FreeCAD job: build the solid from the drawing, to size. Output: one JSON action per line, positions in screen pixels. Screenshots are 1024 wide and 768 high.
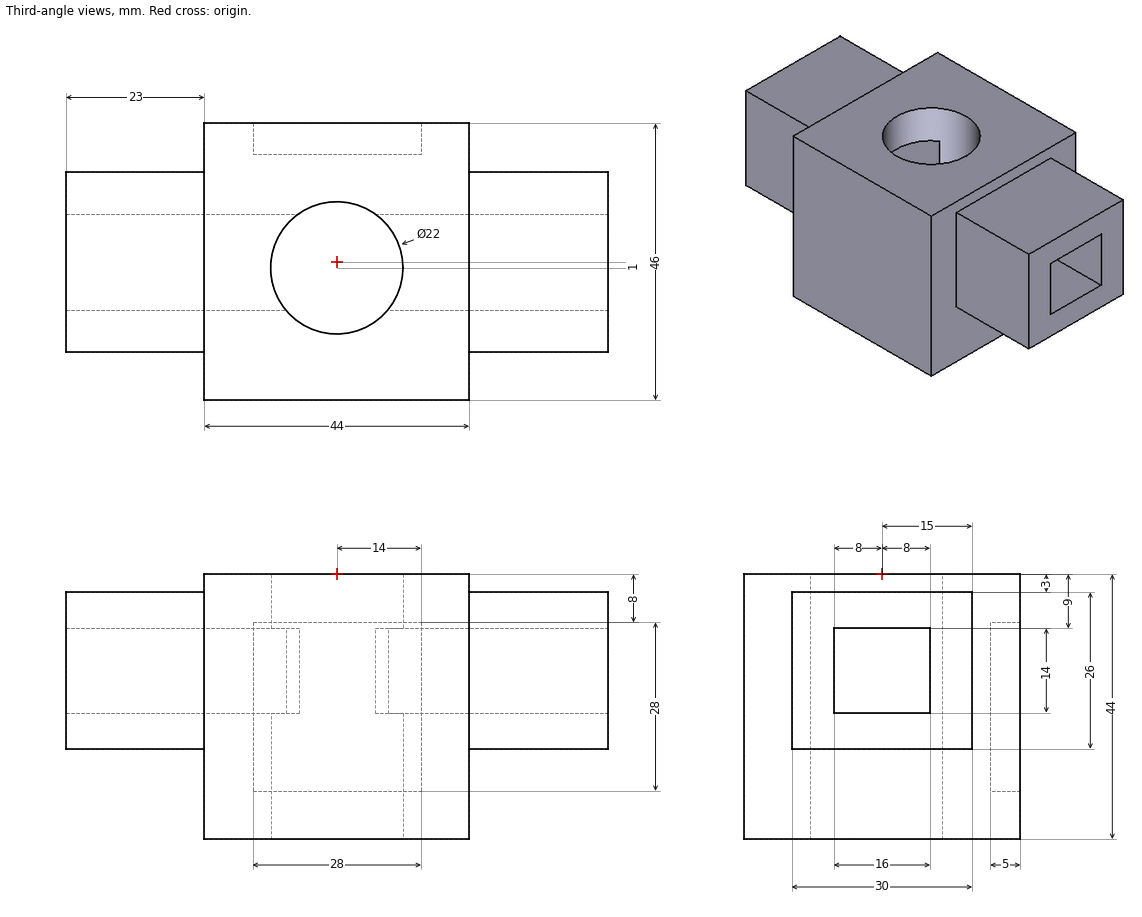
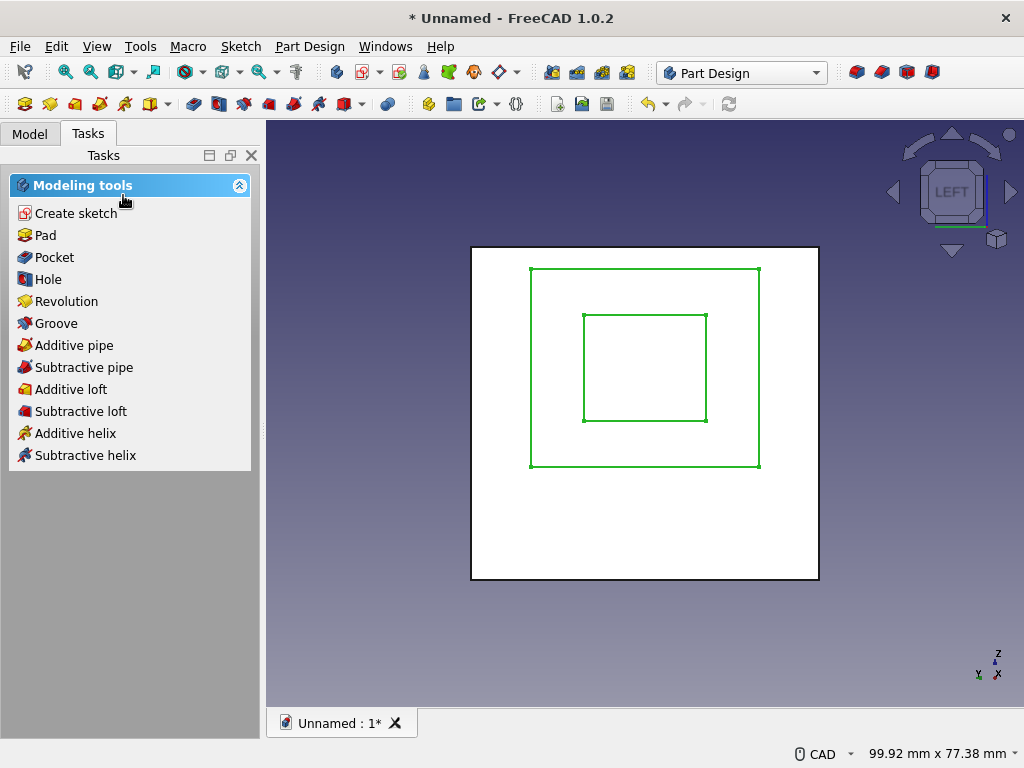
{"action": "left_click", "coordinate": [25, 104]}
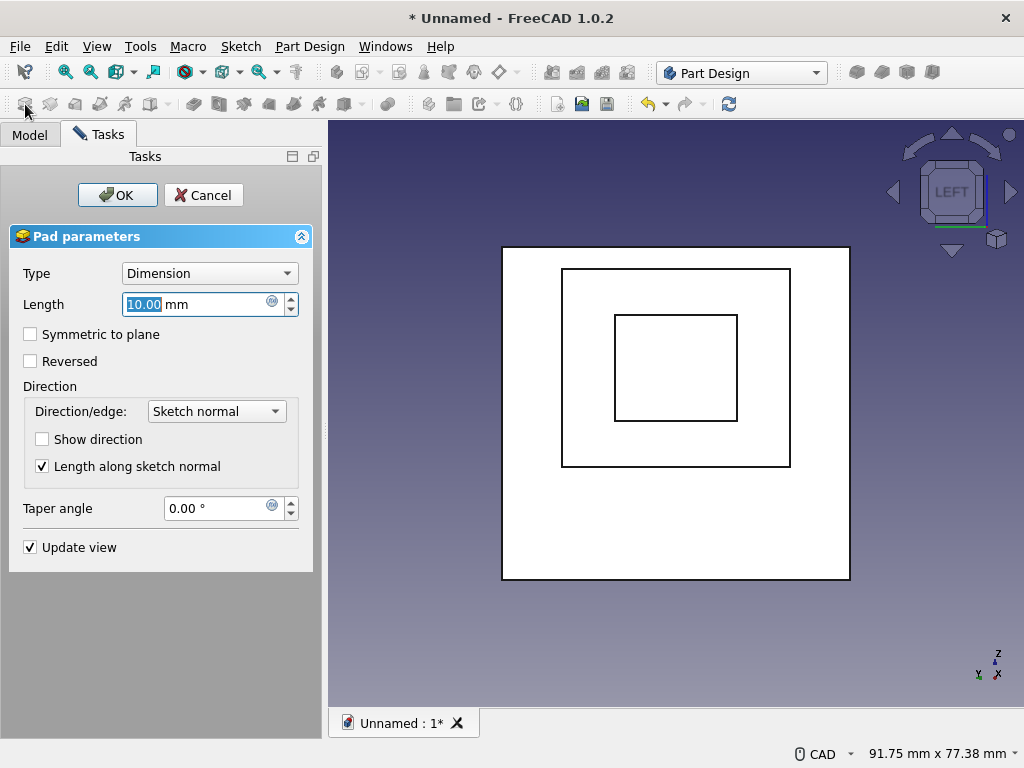
{"action": "type", "text": "23"}
{"action": "key", "text": "Tab"}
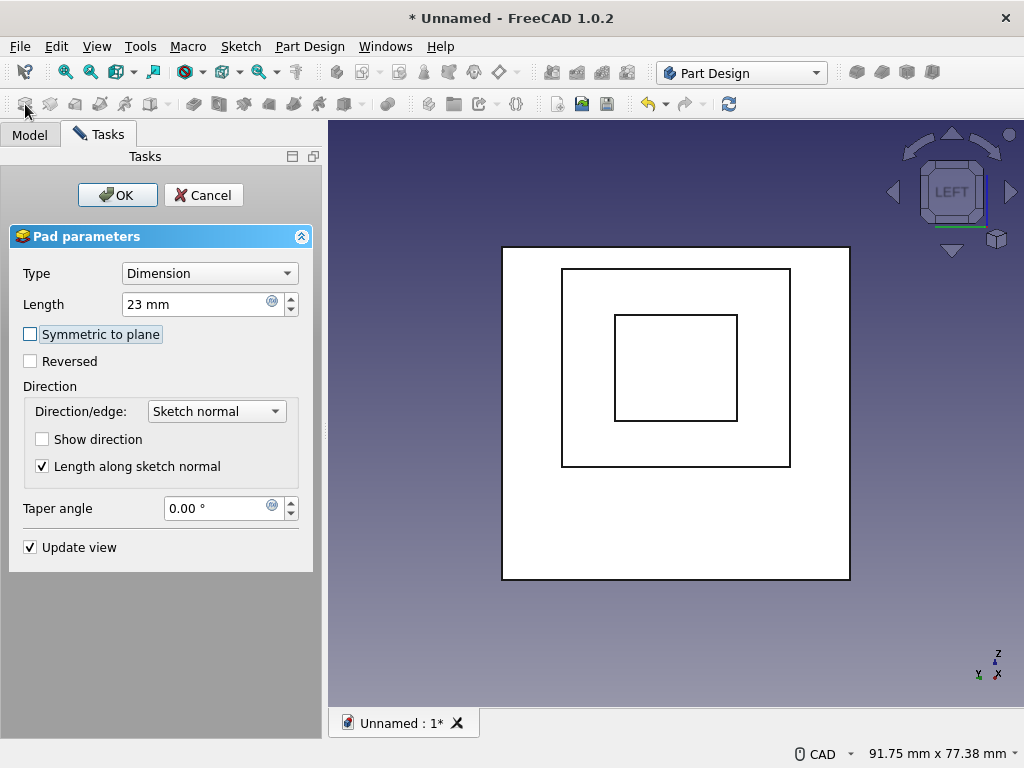
{"action": "left_click", "coordinate": [118, 195]}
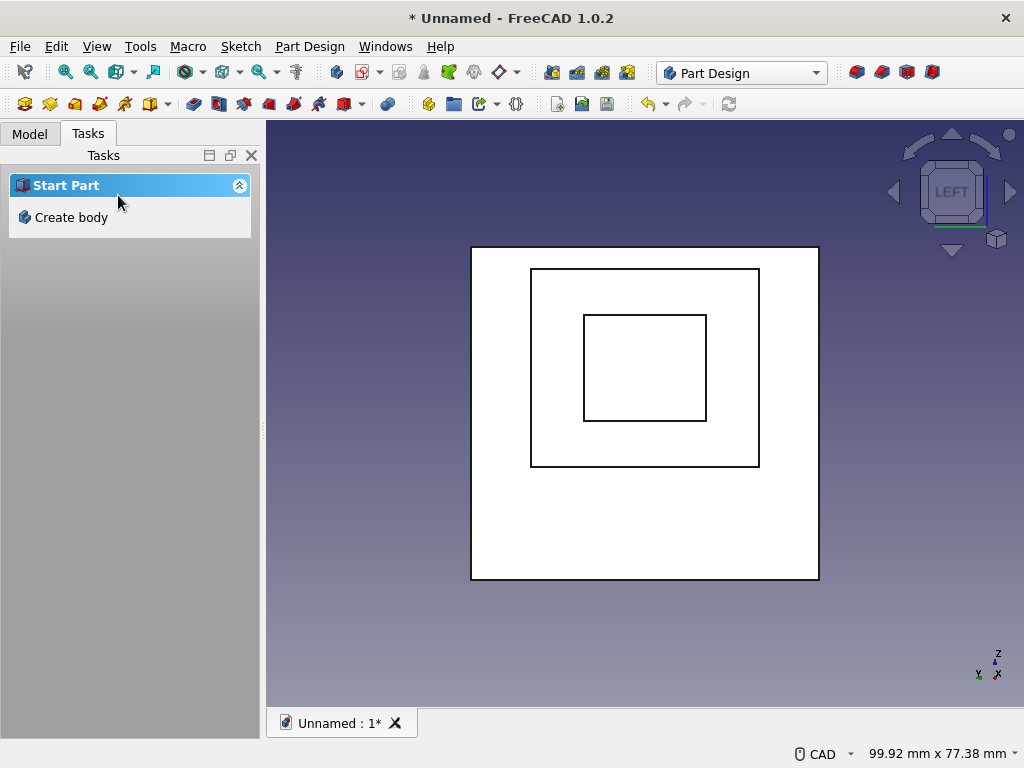
{"action": "left_click", "coordinate": [30, 134]}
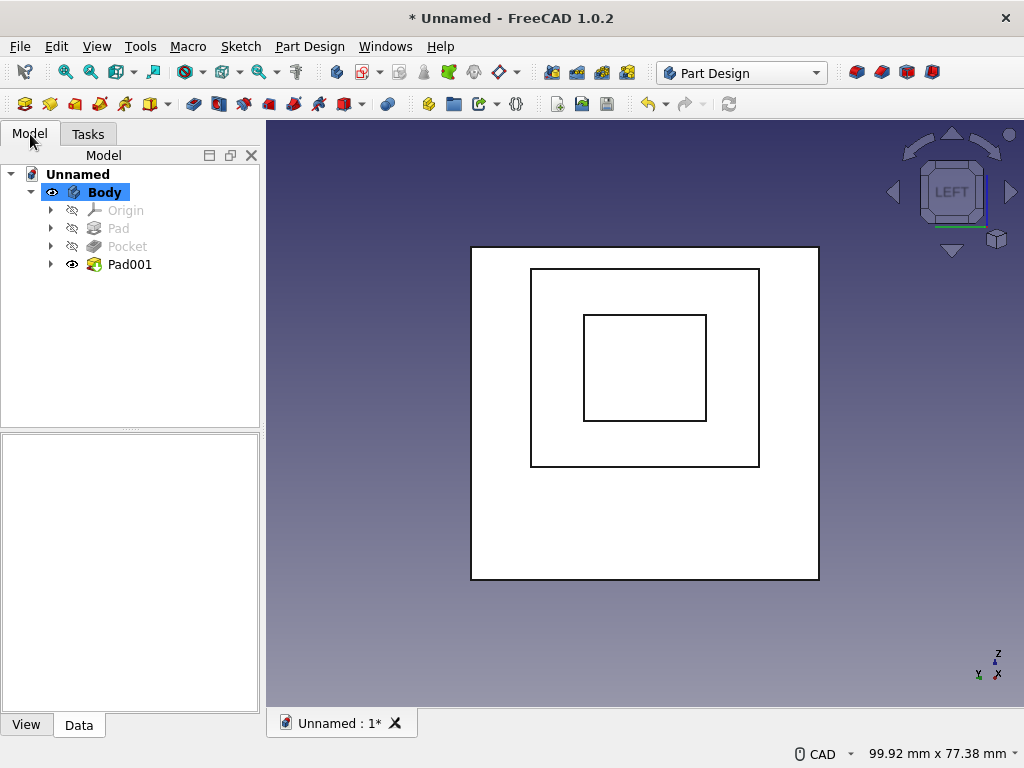
{"action": "left_click", "coordinate": [117, 264]}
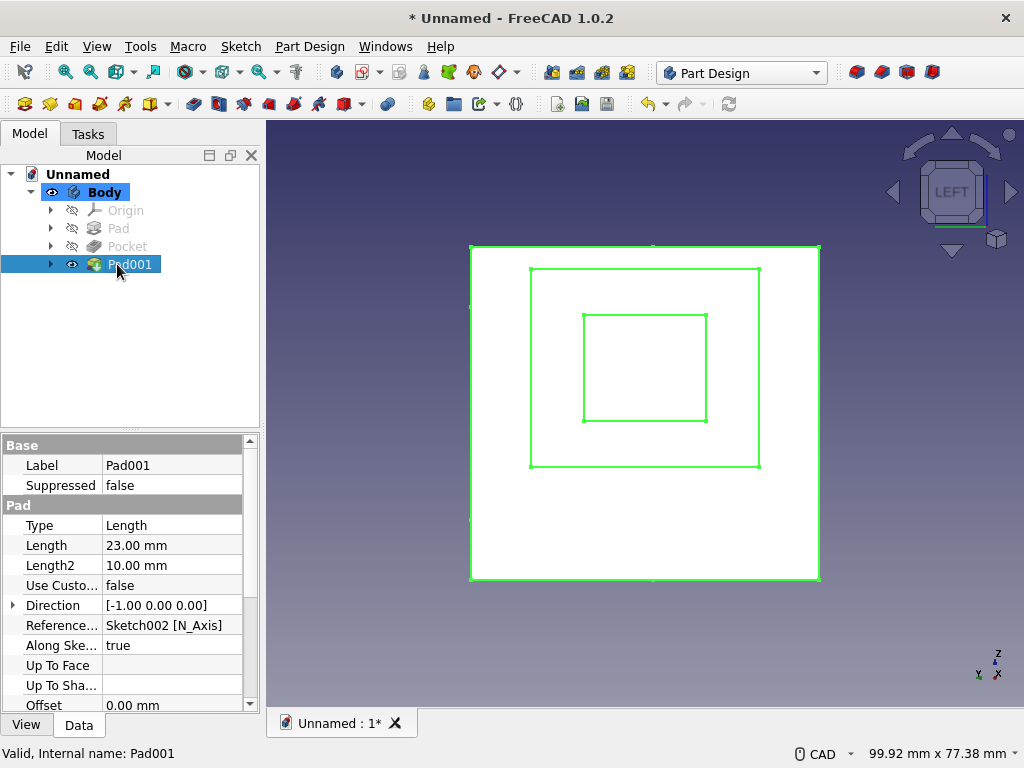
{"action": "left_click", "coordinate": [552, 72]}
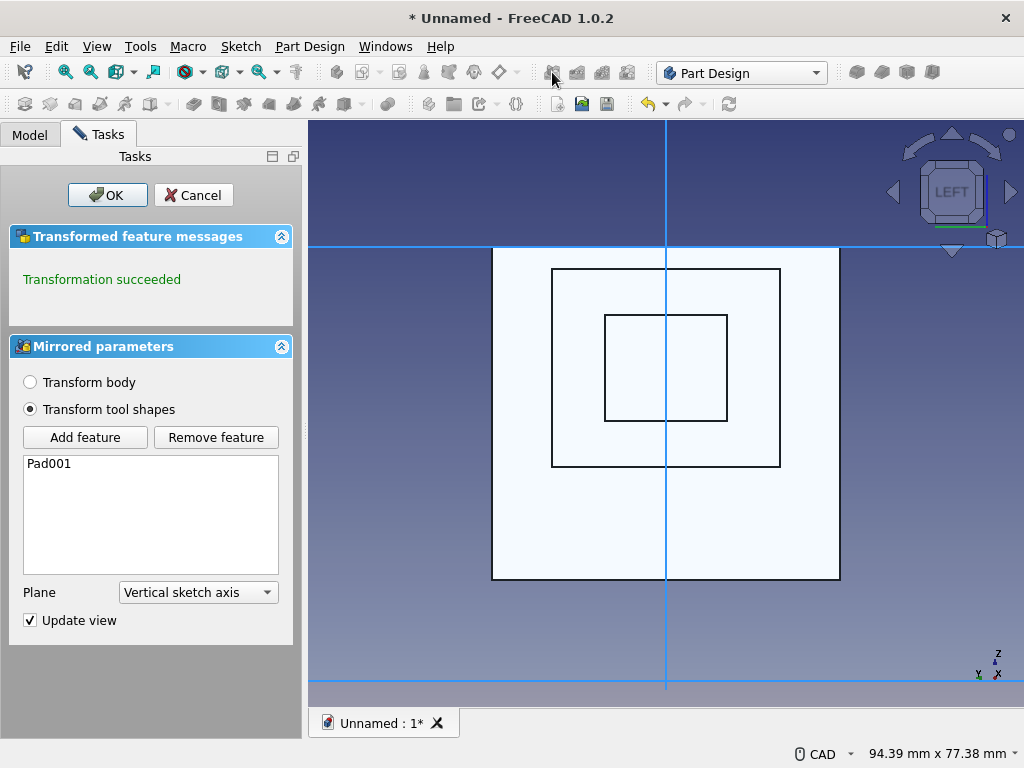
{"action": "left_click", "coordinate": [199, 592]}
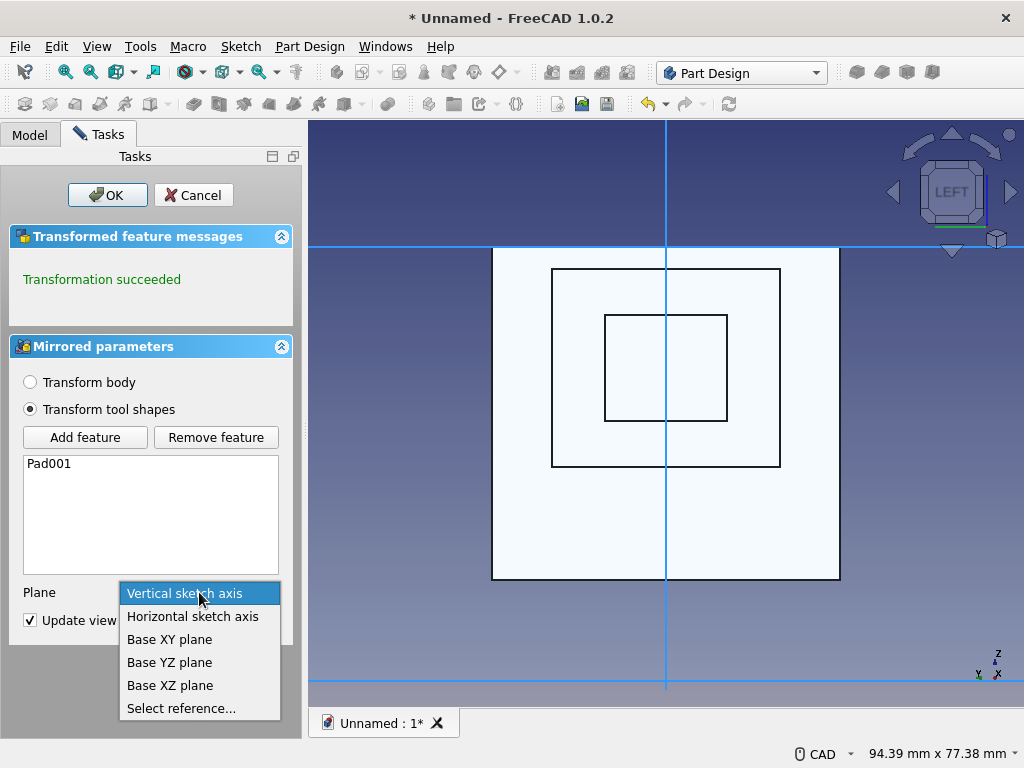
{"action": "left_click", "coordinate": [198, 662]}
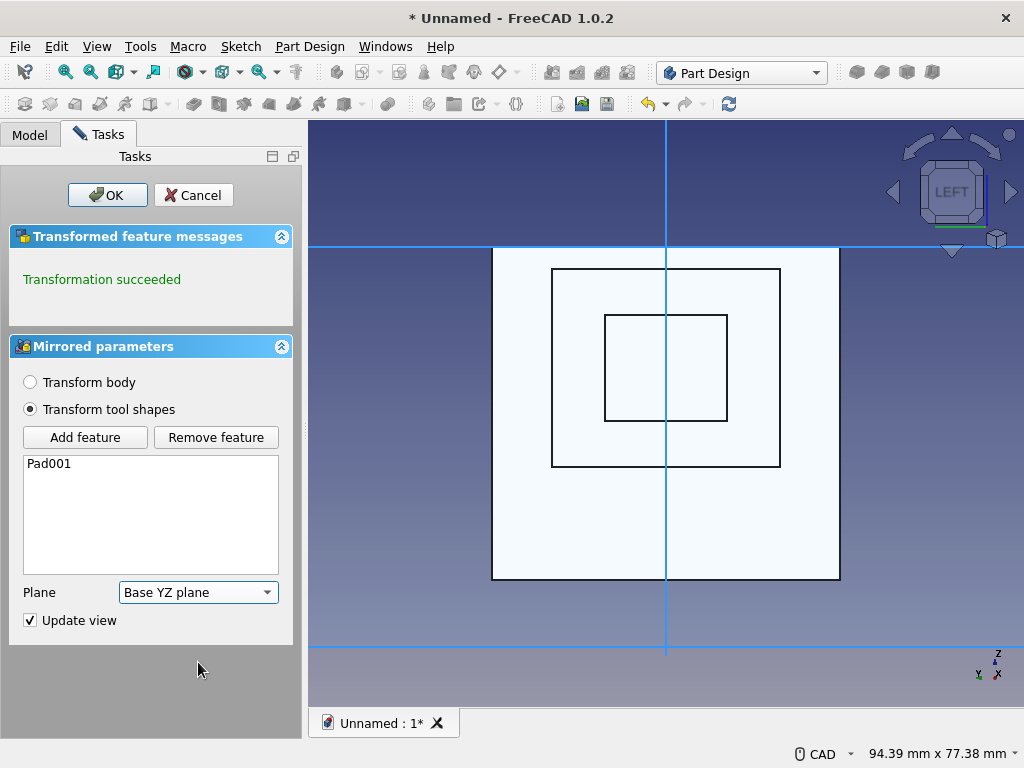
{"action": "left_click", "coordinate": [108, 195]}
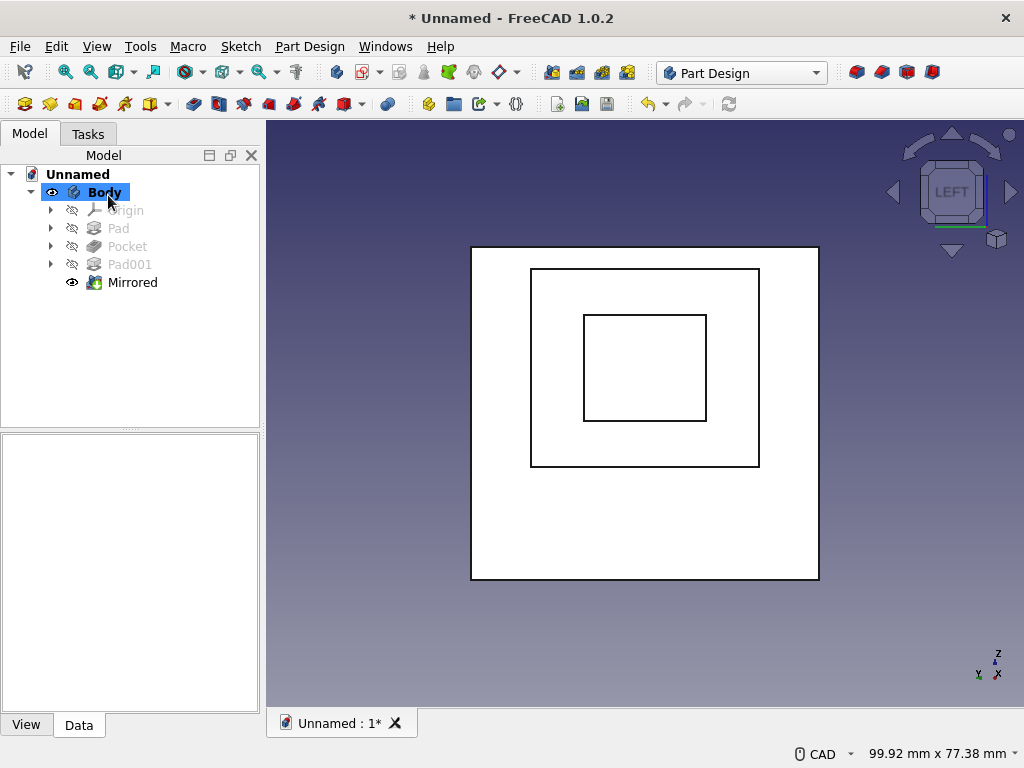
{"action": "key", "text": "0"}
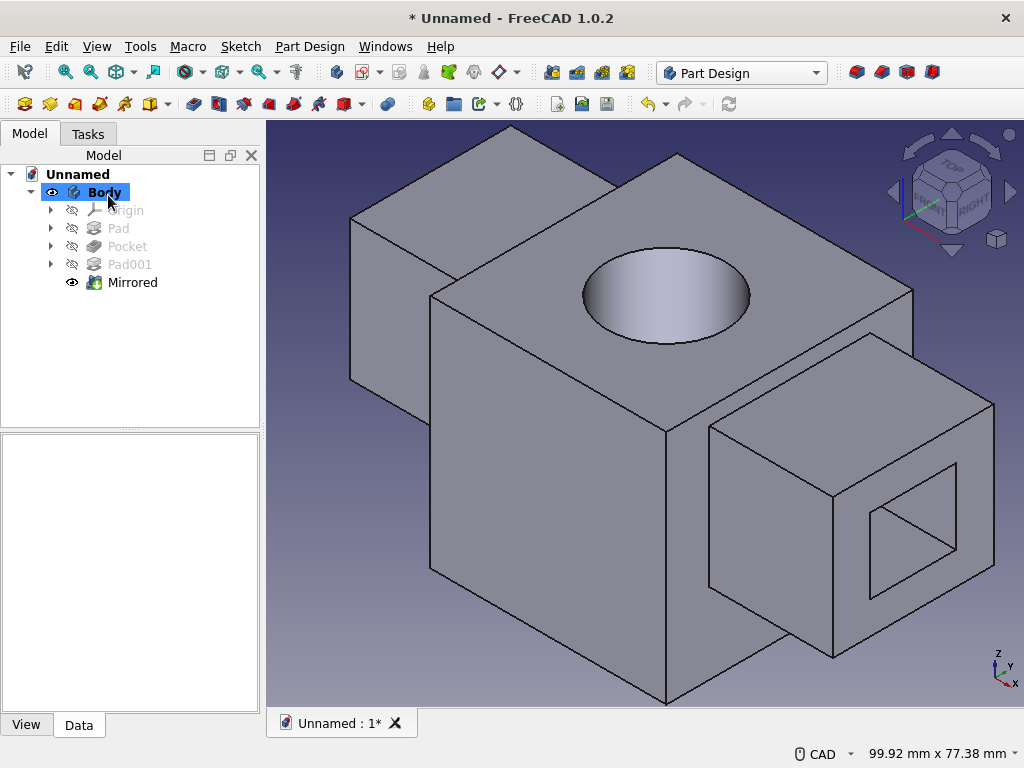
{"action": "left_click", "coordinate": [66, 72]}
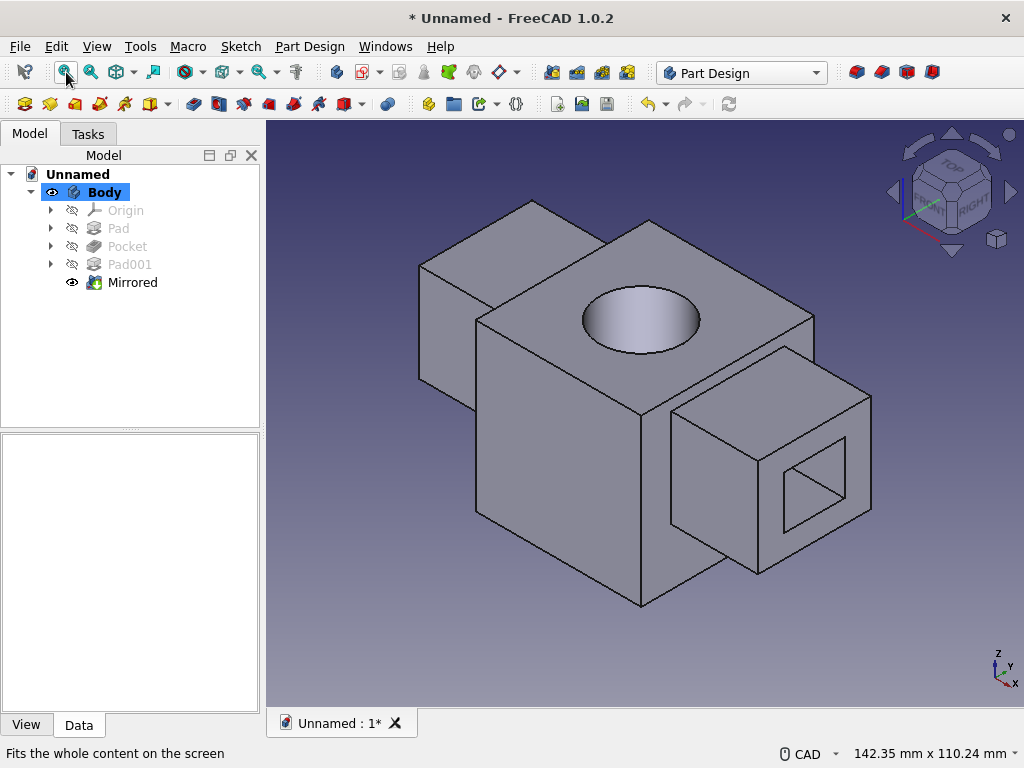
{"action": "left_click", "coordinate": [863, 424]}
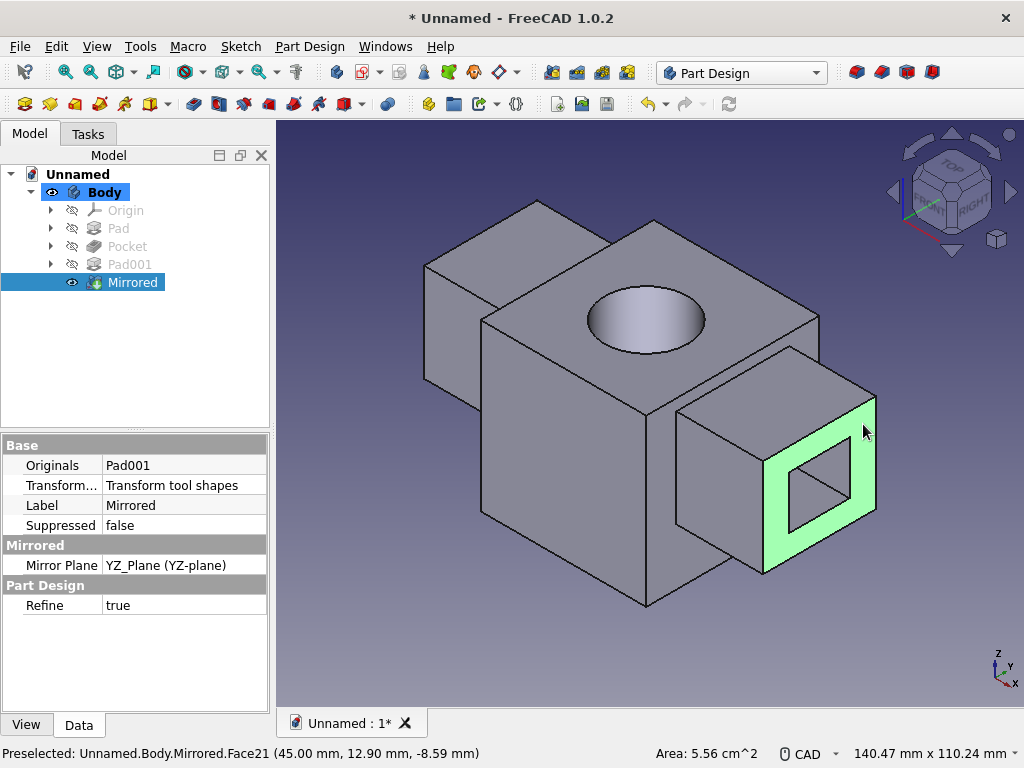
{"action": "left_click", "coordinate": [362, 72]}